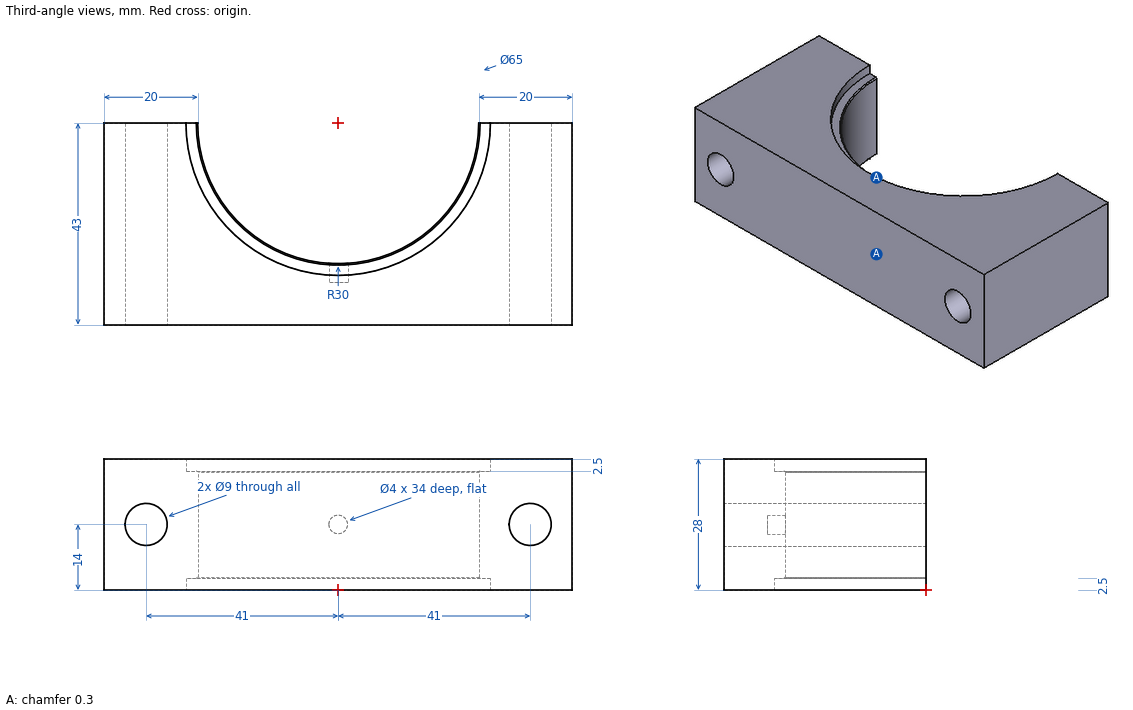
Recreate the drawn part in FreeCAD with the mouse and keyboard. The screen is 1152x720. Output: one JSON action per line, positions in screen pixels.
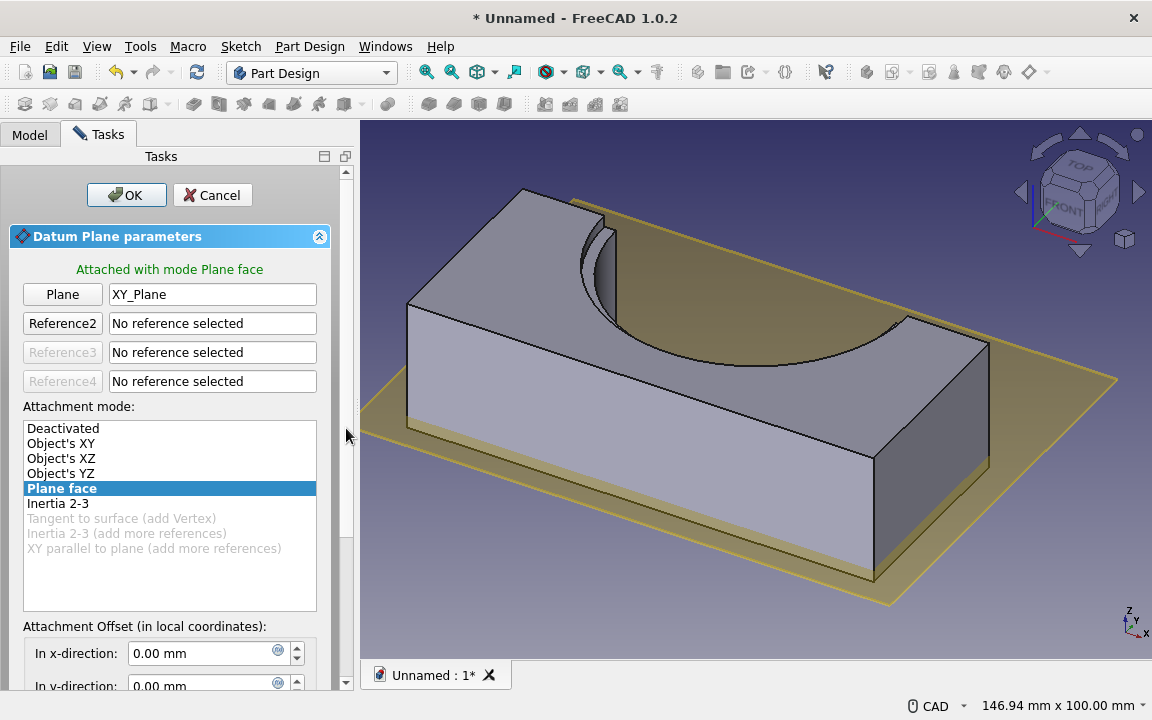
{"action": "left_click", "coordinate": [127, 195]}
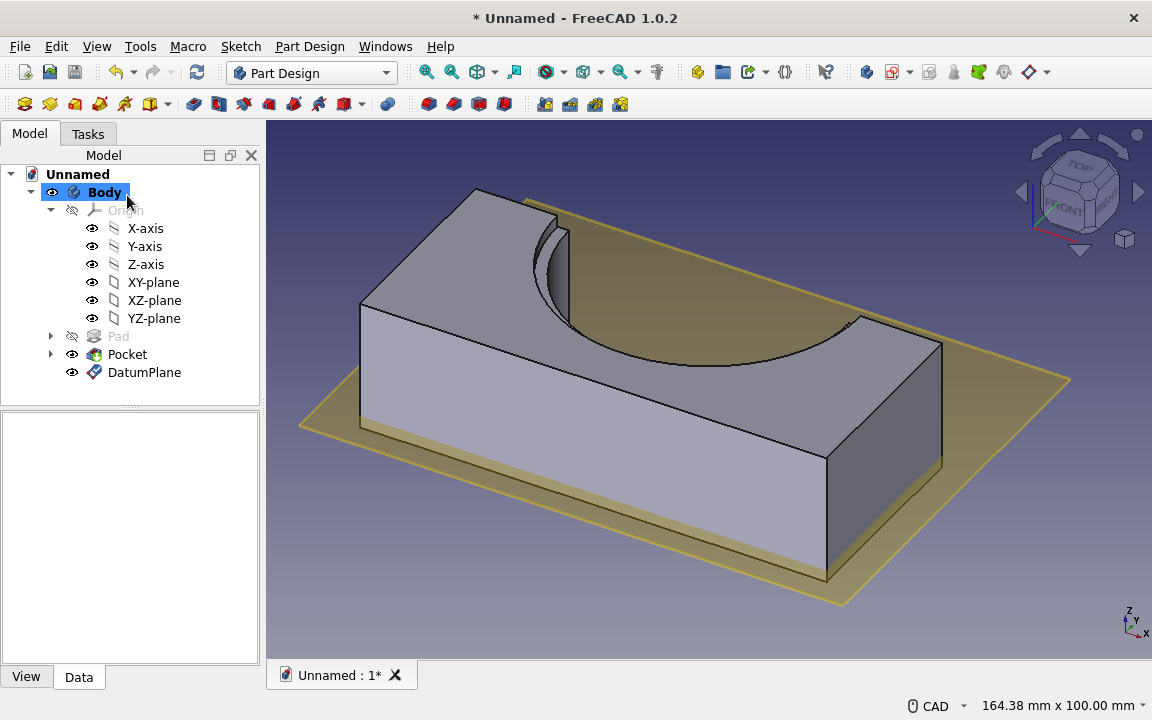
{"action": "left_click", "coordinate": [117, 372]}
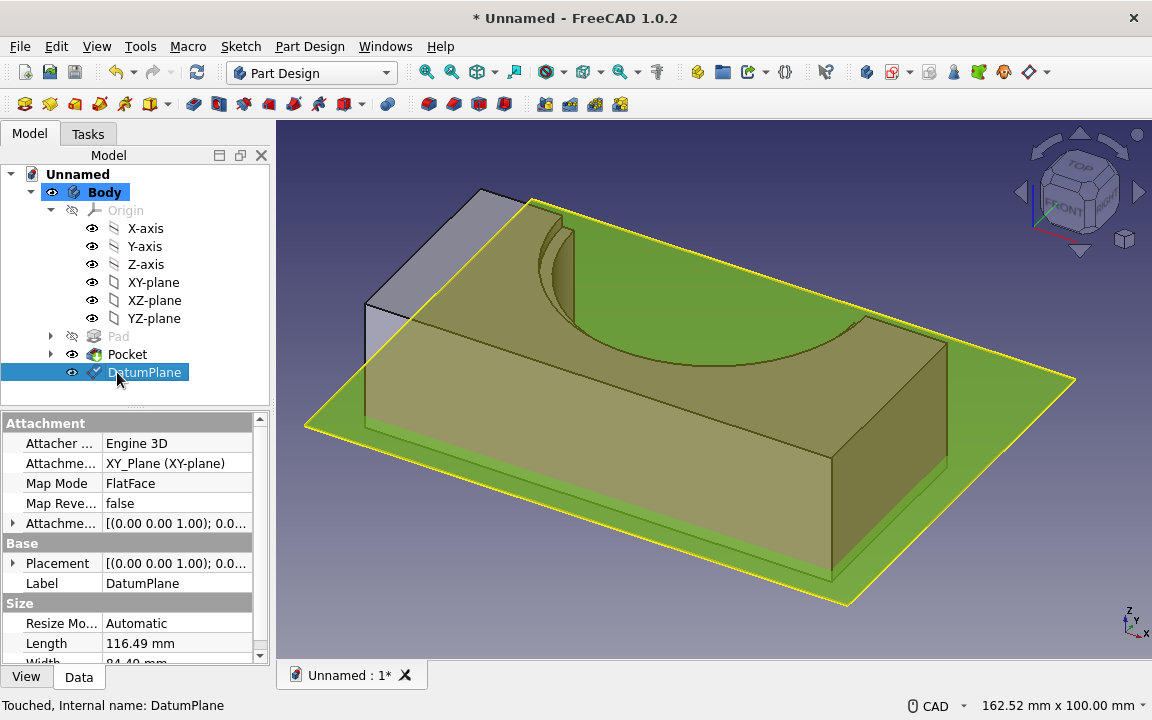
{"action": "left_click", "coordinate": [892, 72]}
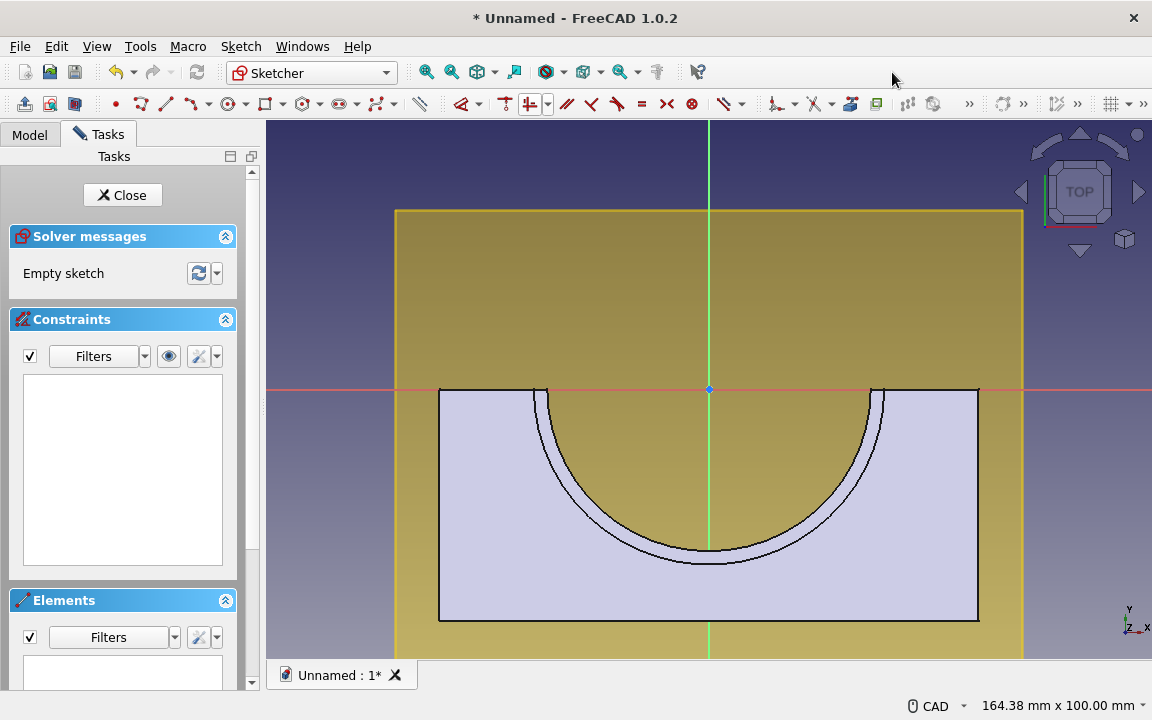
{"action": "left_click", "coordinate": [75, 104]}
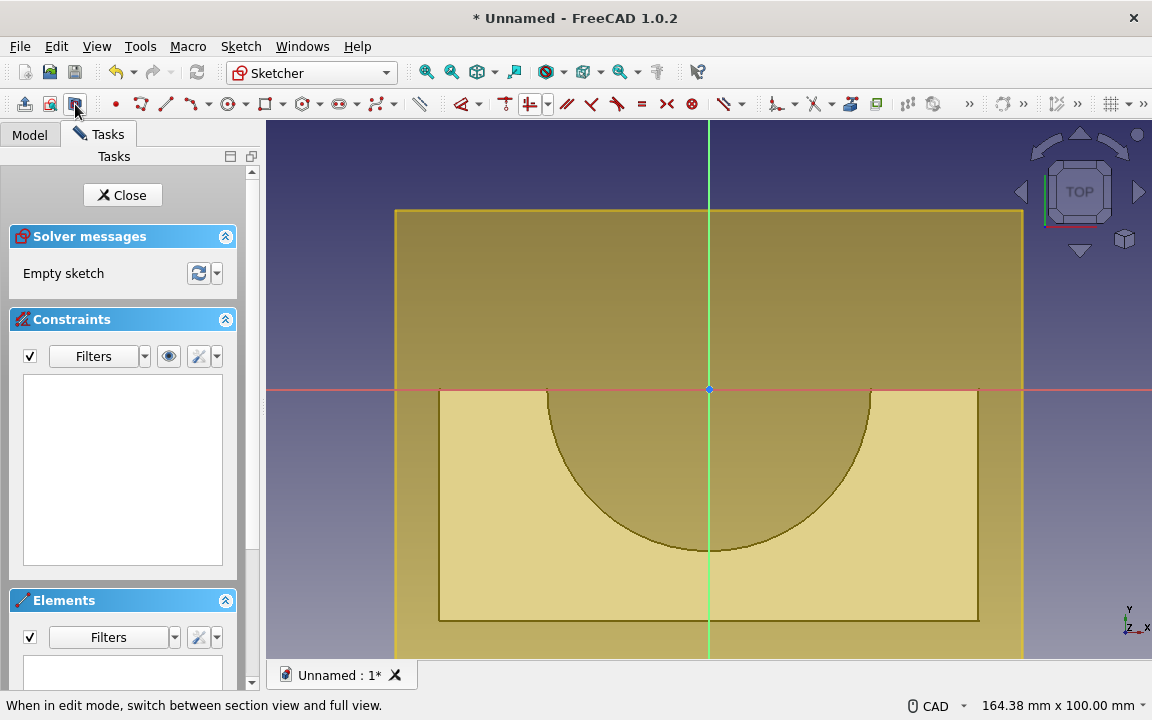
{"action": "left_click", "coordinate": [228, 104]}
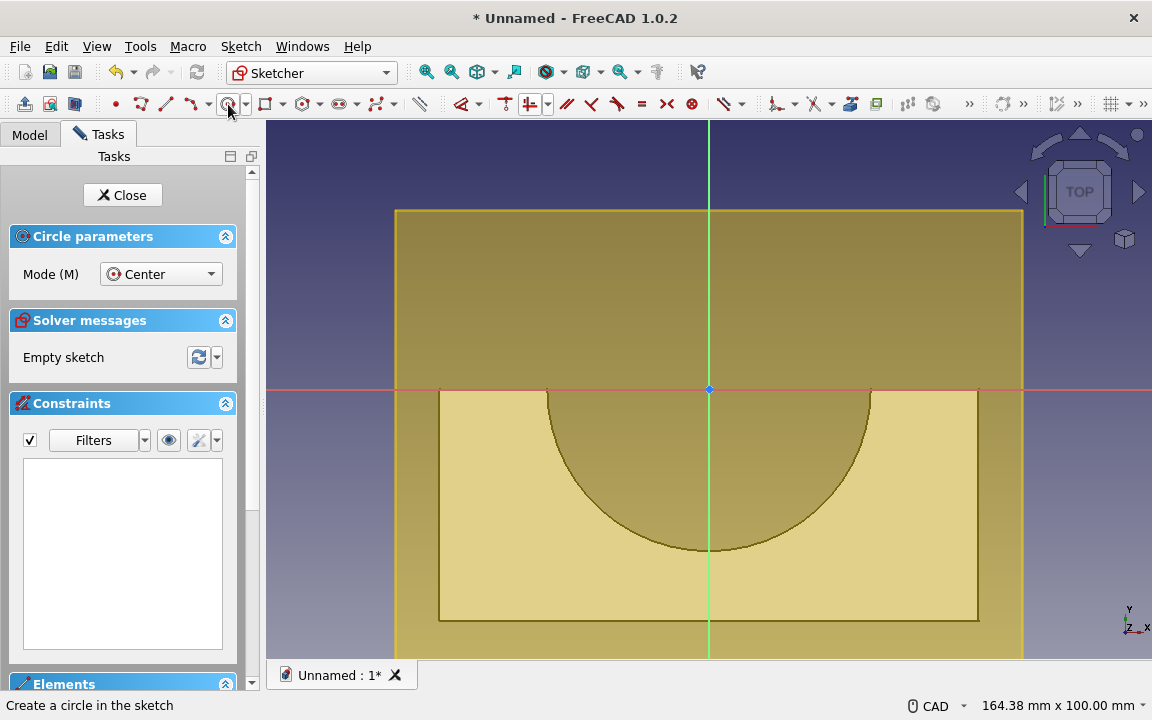
{"action": "left_click", "coordinate": [709, 390]}
{"action": "left_click", "coordinate": [833, 266]}
{"action": "key", "text": "Escape"}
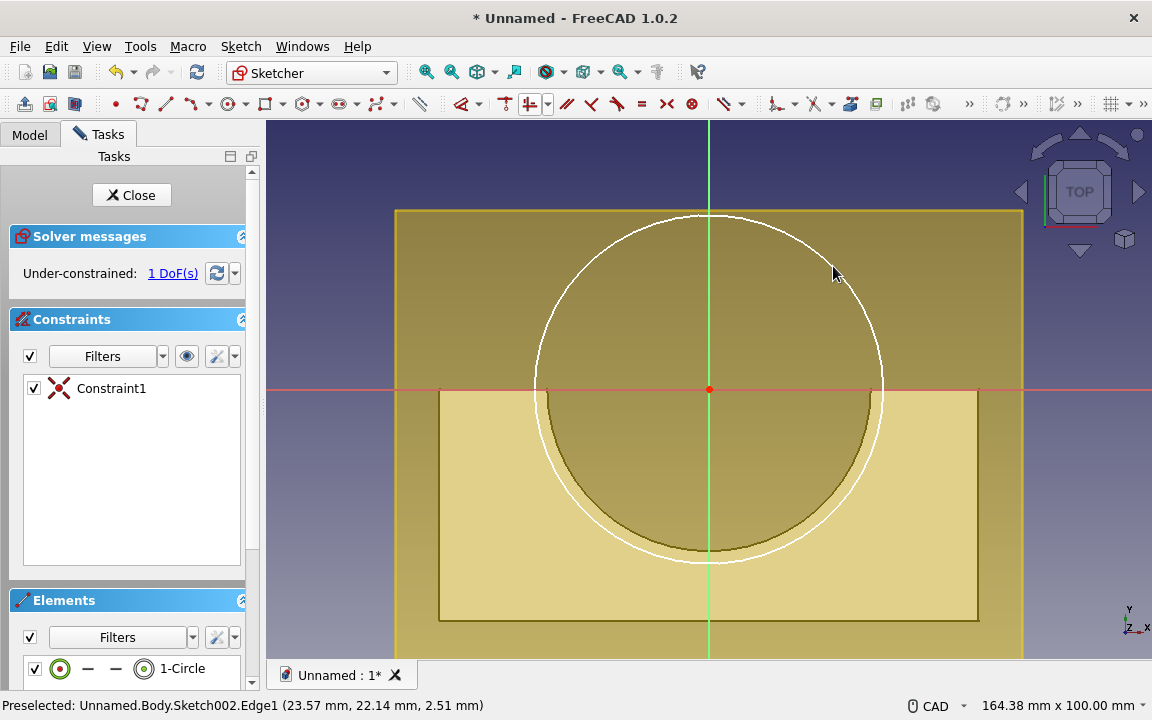
{"action": "left_click", "coordinate": [460, 104]}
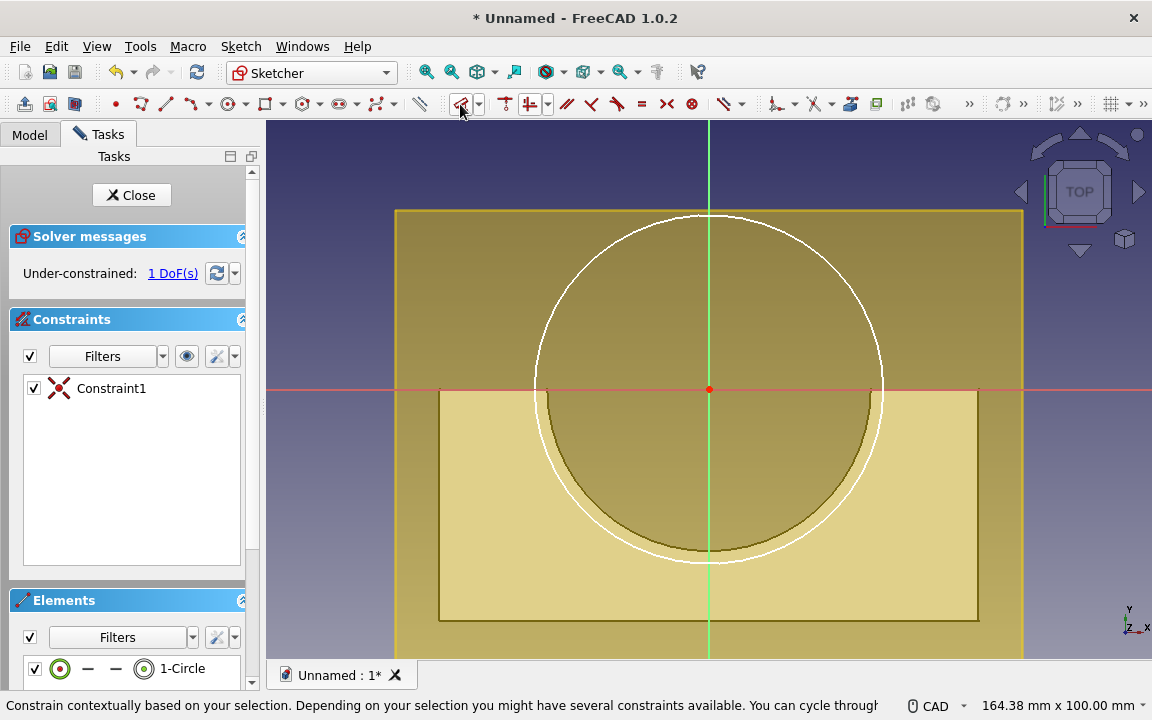
{"action": "left_click", "coordinate": [832, 266]}
{"action": "left_click", "coordinate": [855, 243]}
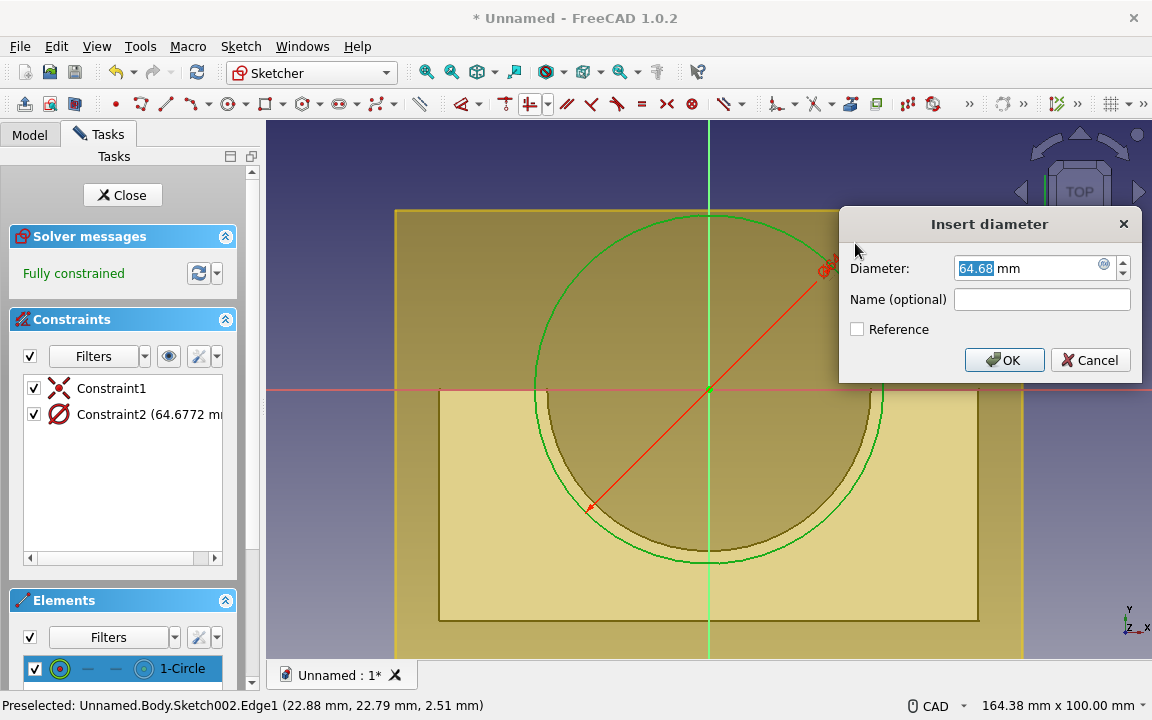
{"action": "type", "text": "65"}
{"action": "key", "text": "Return"}
{"action": "key", "text": "Escape"}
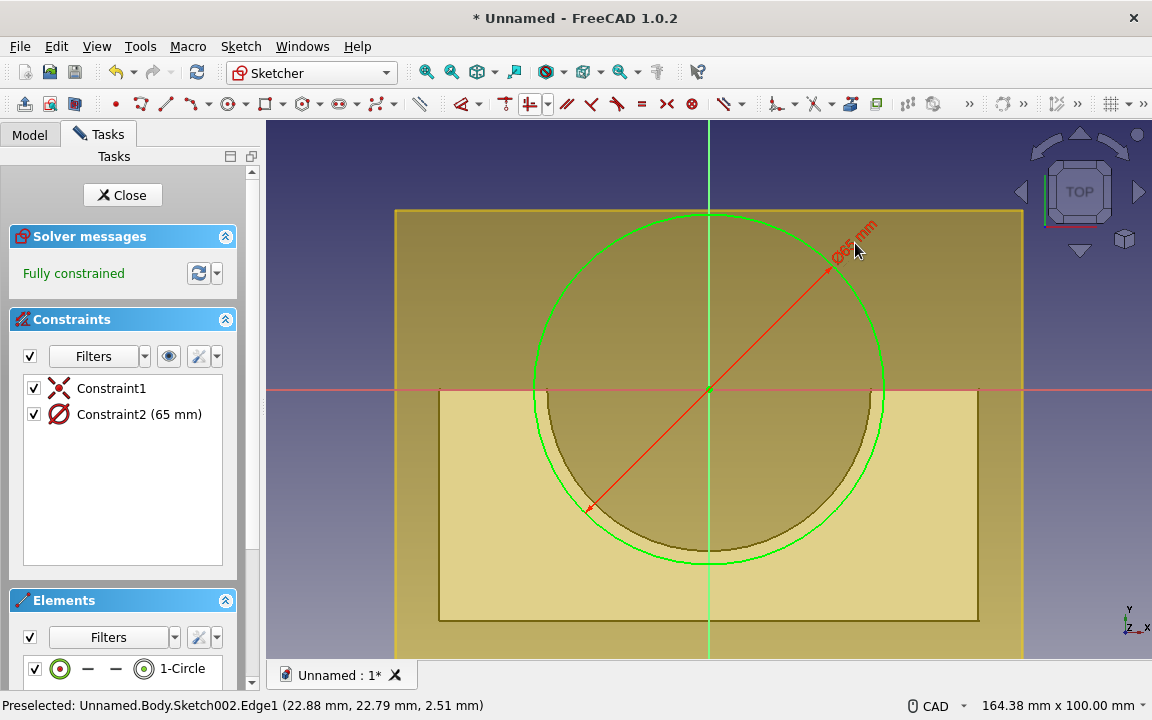
{"action": "left_click", "coordinate": [123, 195]}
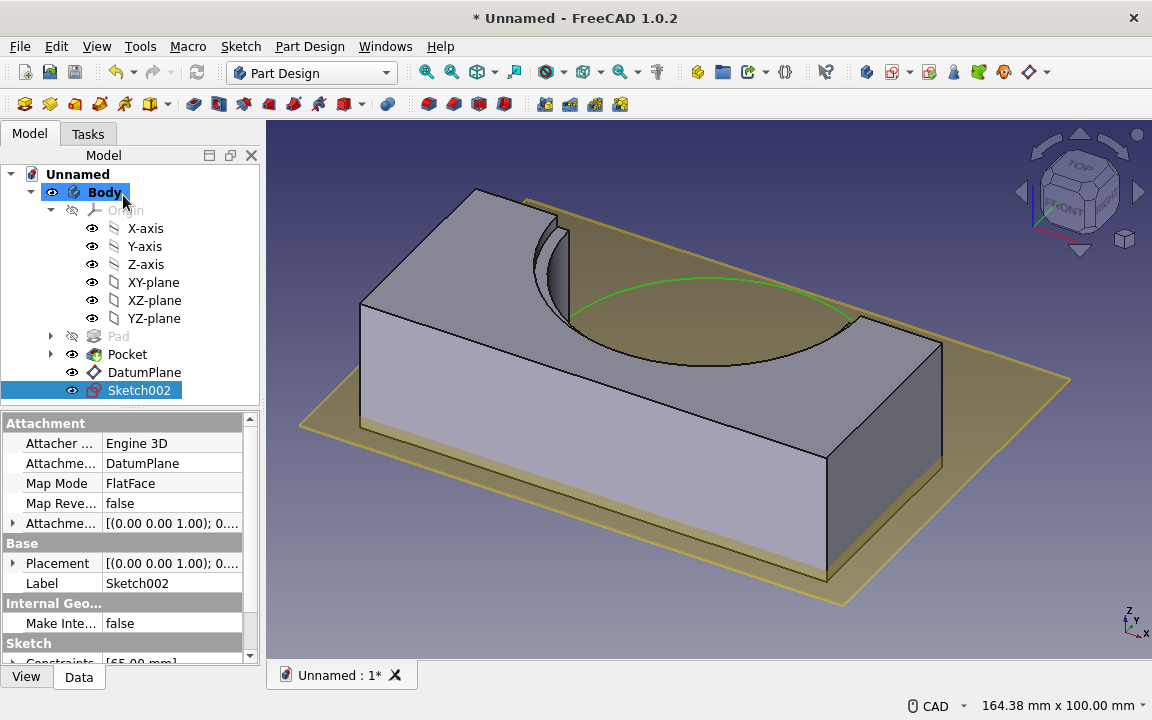
{"action": "left_click", "coordinate": [194, 104]}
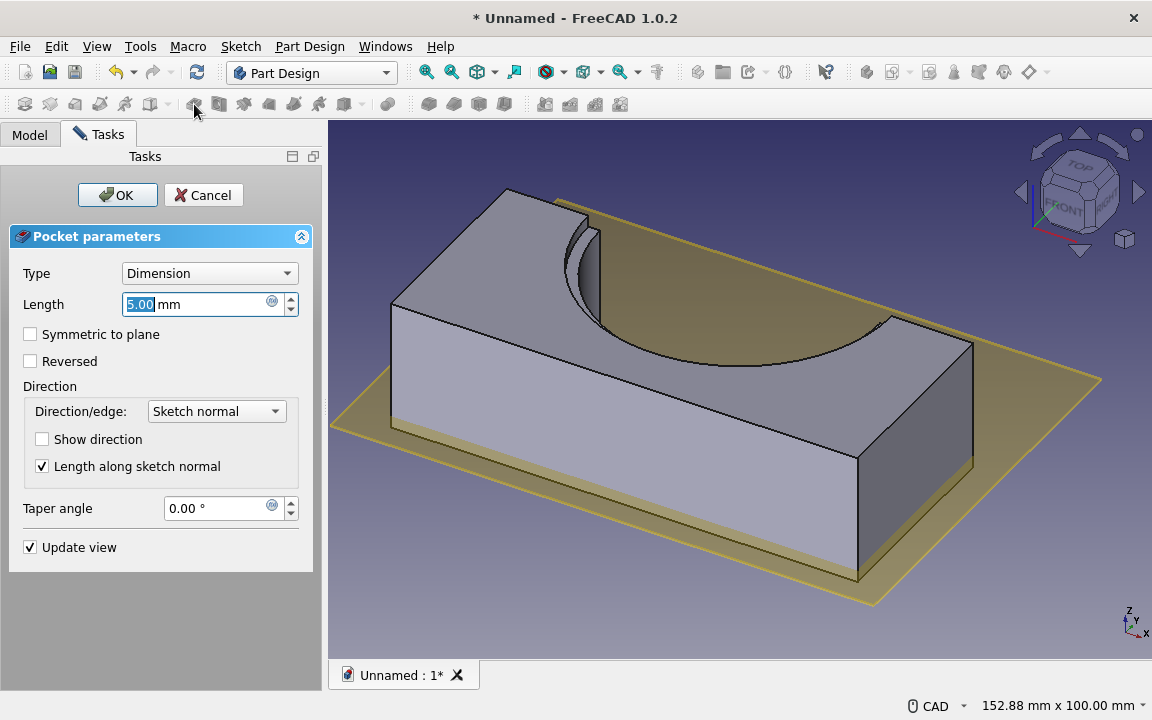
{"action": "type", "text": "2.5"}
{"action": "key", "text": "Tab"}